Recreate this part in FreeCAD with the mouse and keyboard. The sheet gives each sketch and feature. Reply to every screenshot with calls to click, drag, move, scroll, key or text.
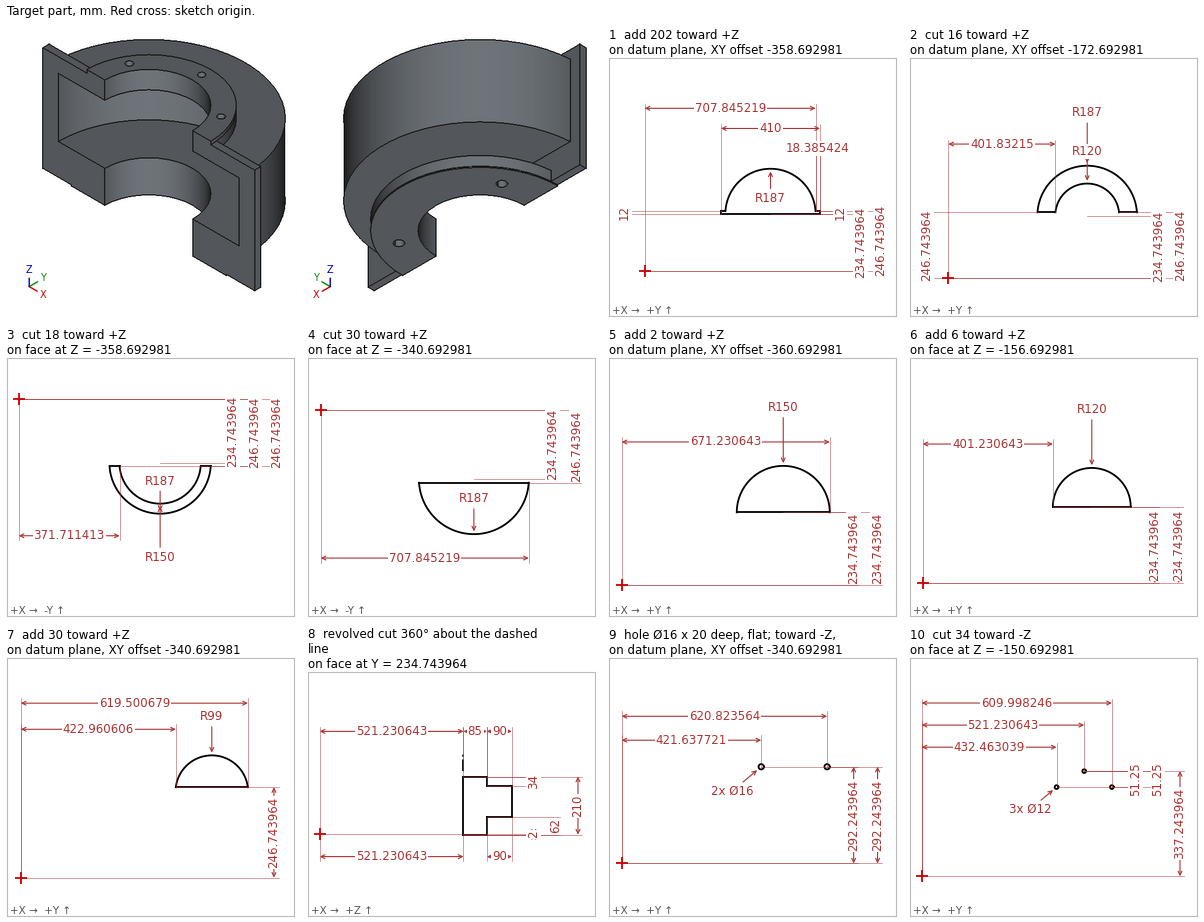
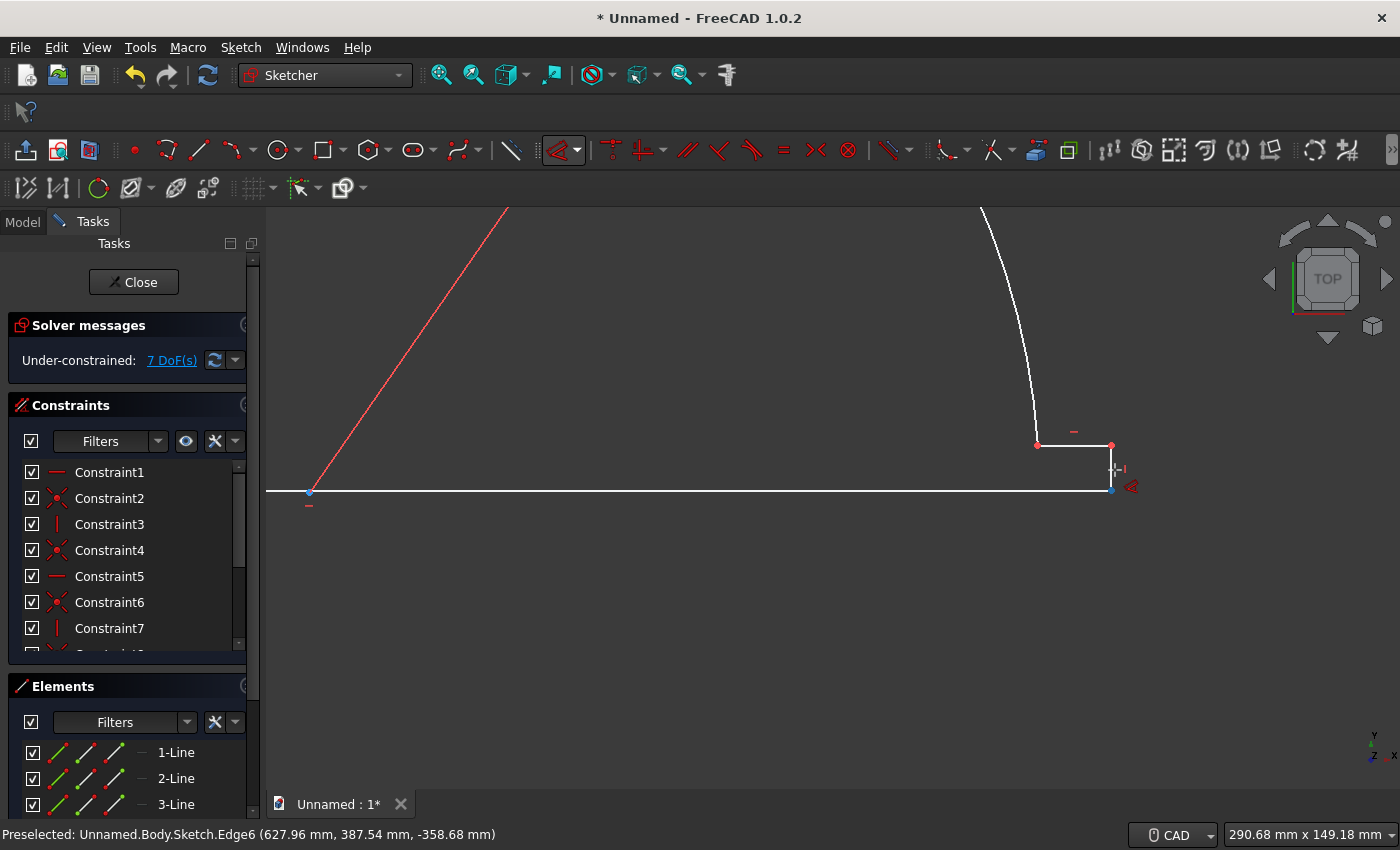
click(1111, 468)
click(1145, 468)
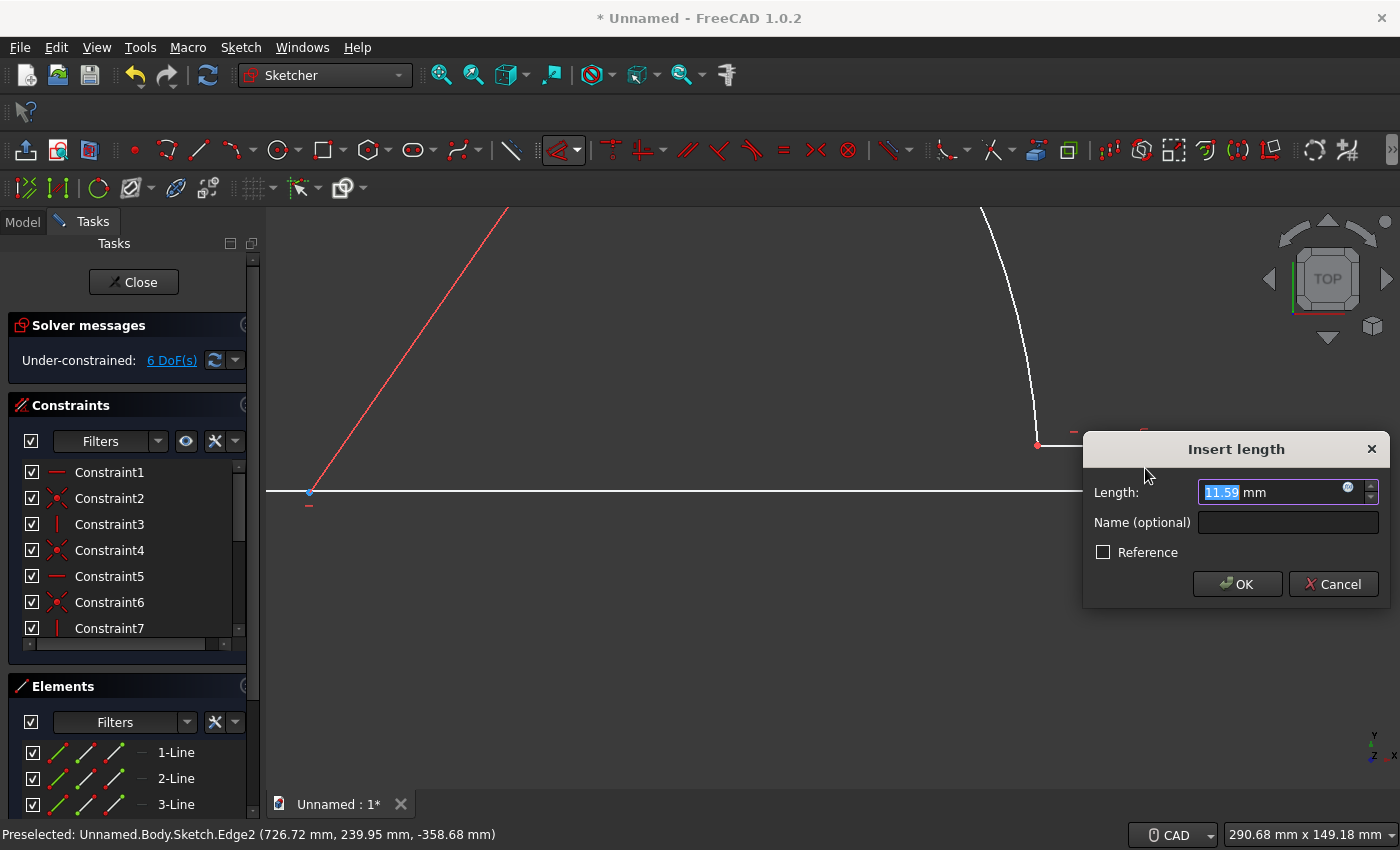
text(12)
key(Return)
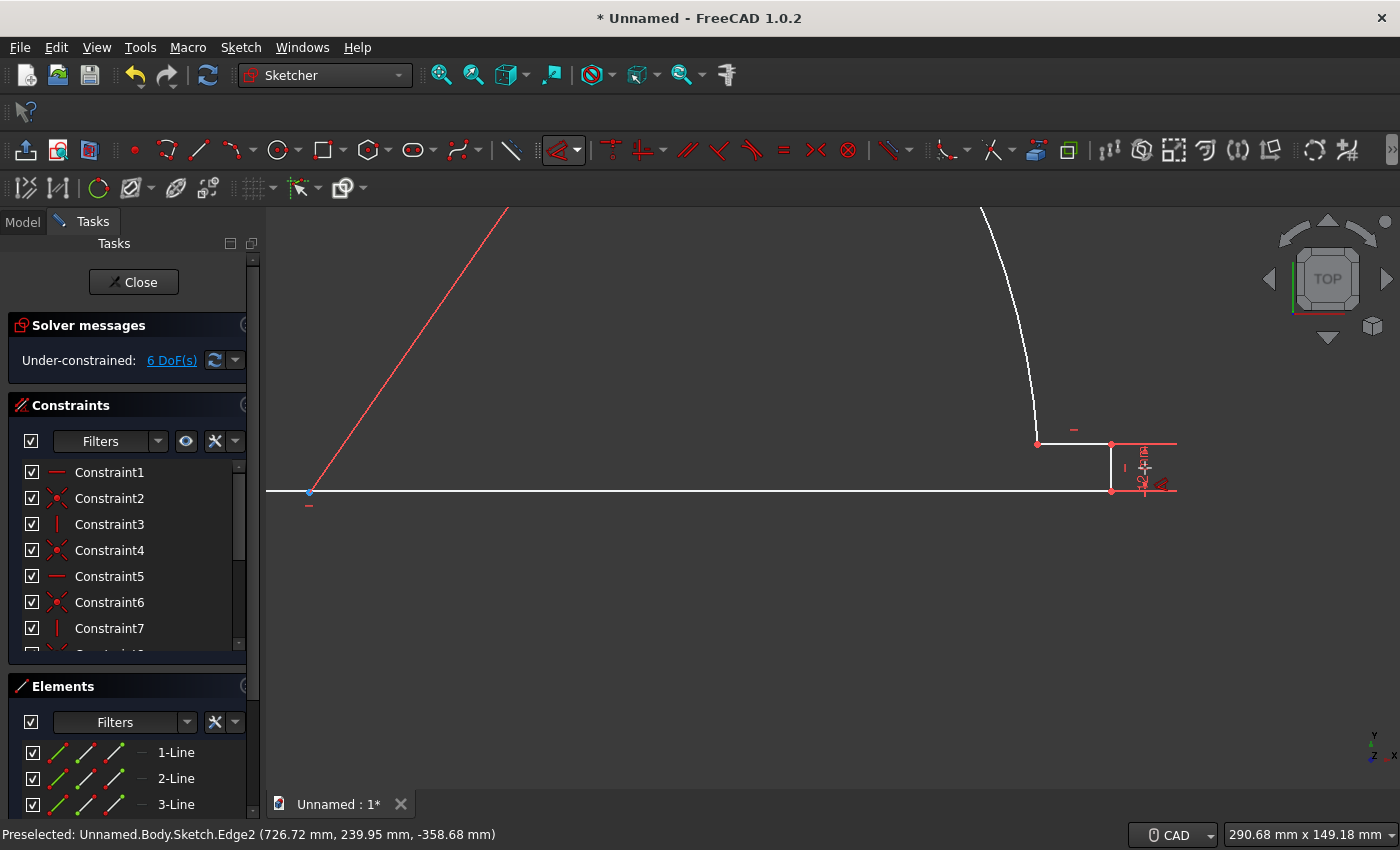
scroll(1115, 470, down, 7)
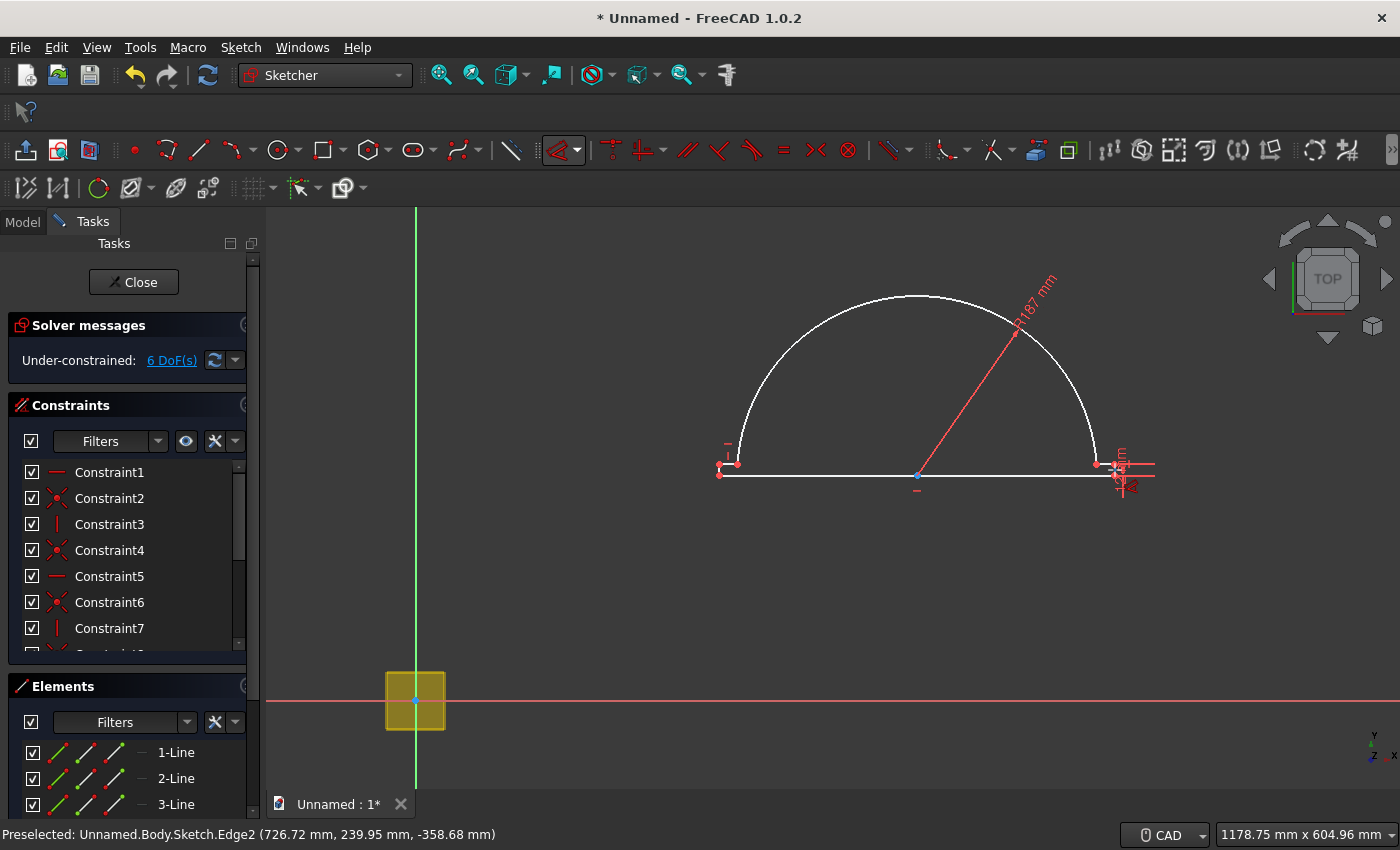
scroll(719, 472, up, 7)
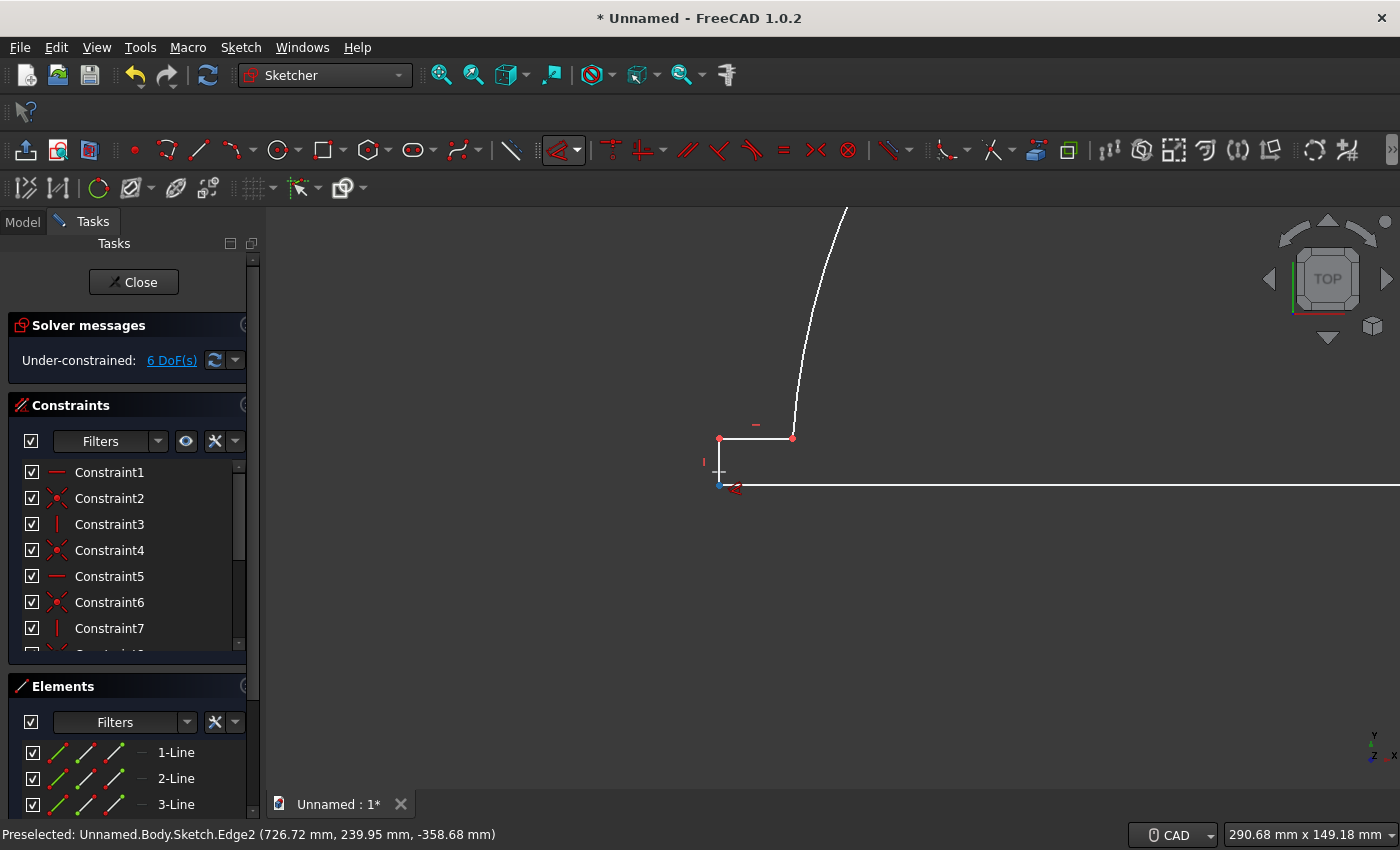
click(719, 471)
click(685, 462)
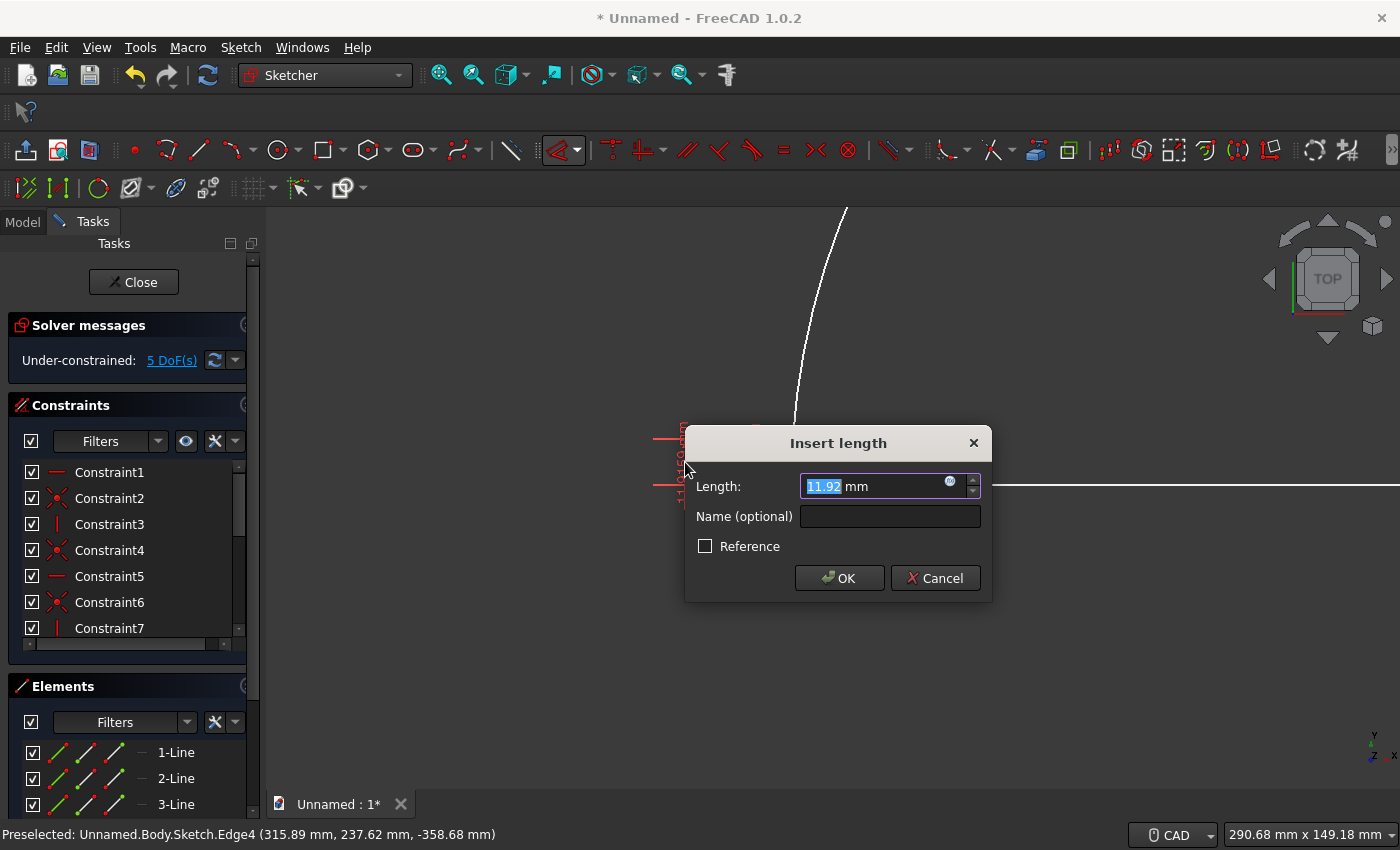
text(12)
key(Return)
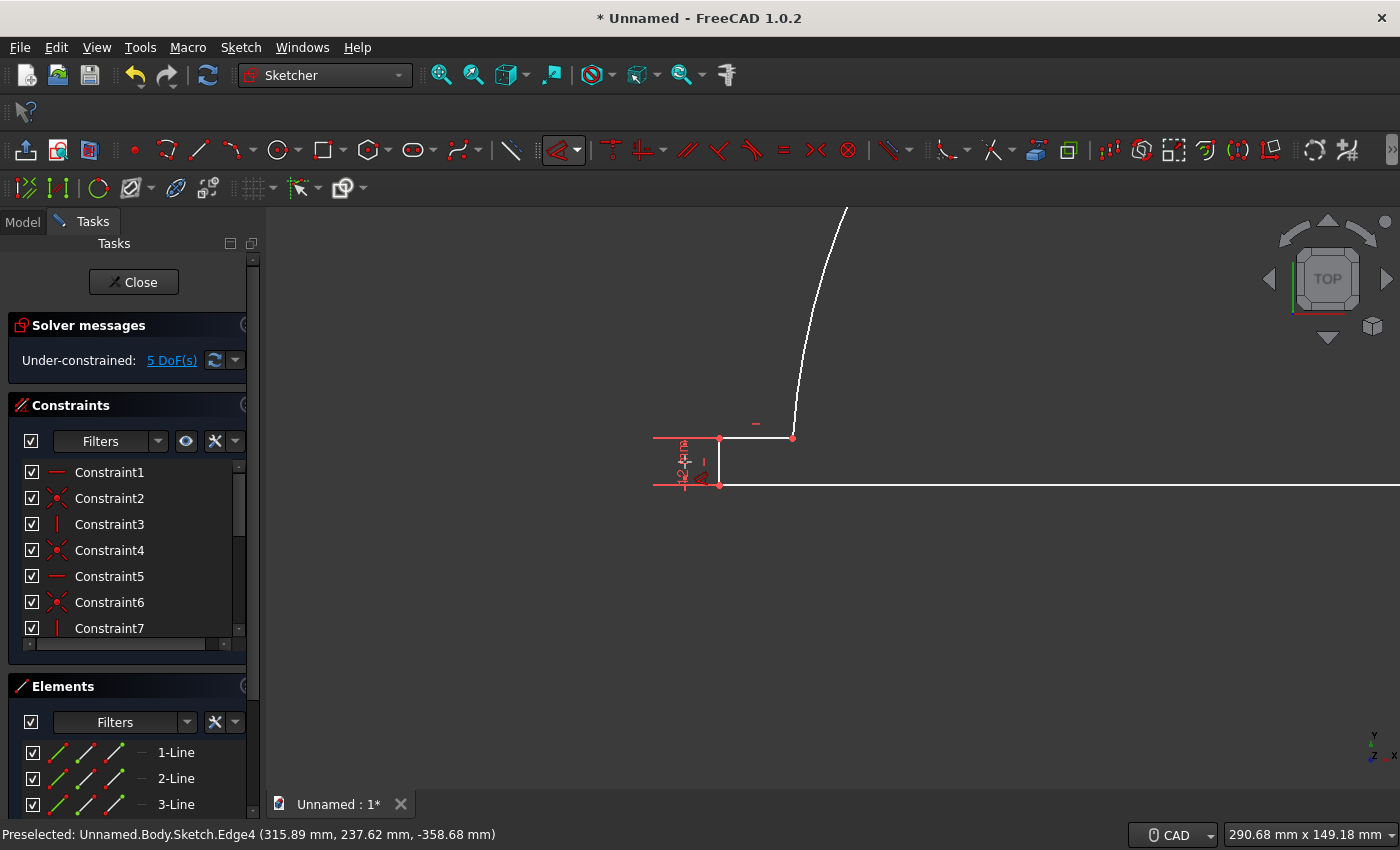
scroll(719, 472, down, 7)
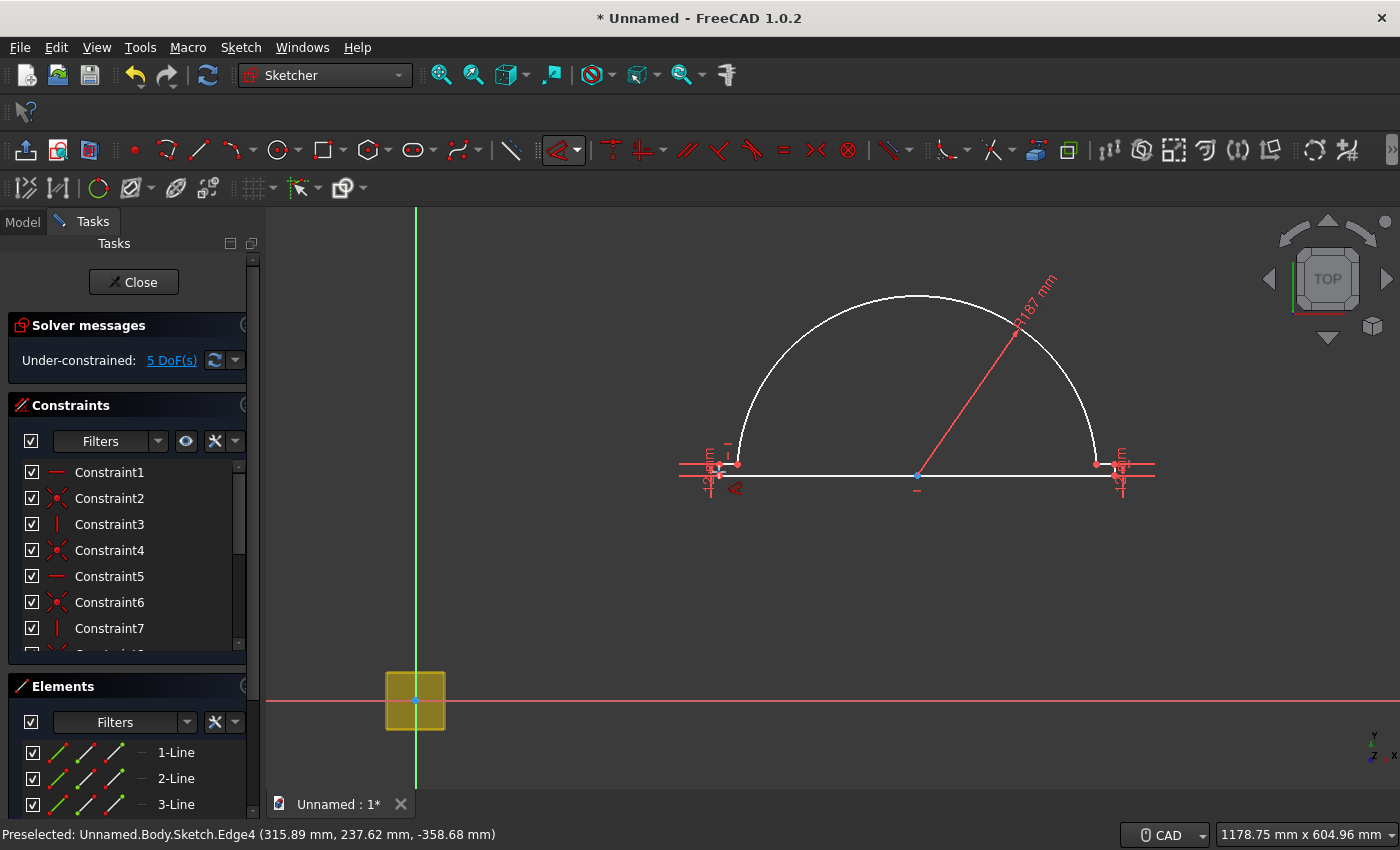
click(838, 476)
click(917, 442)